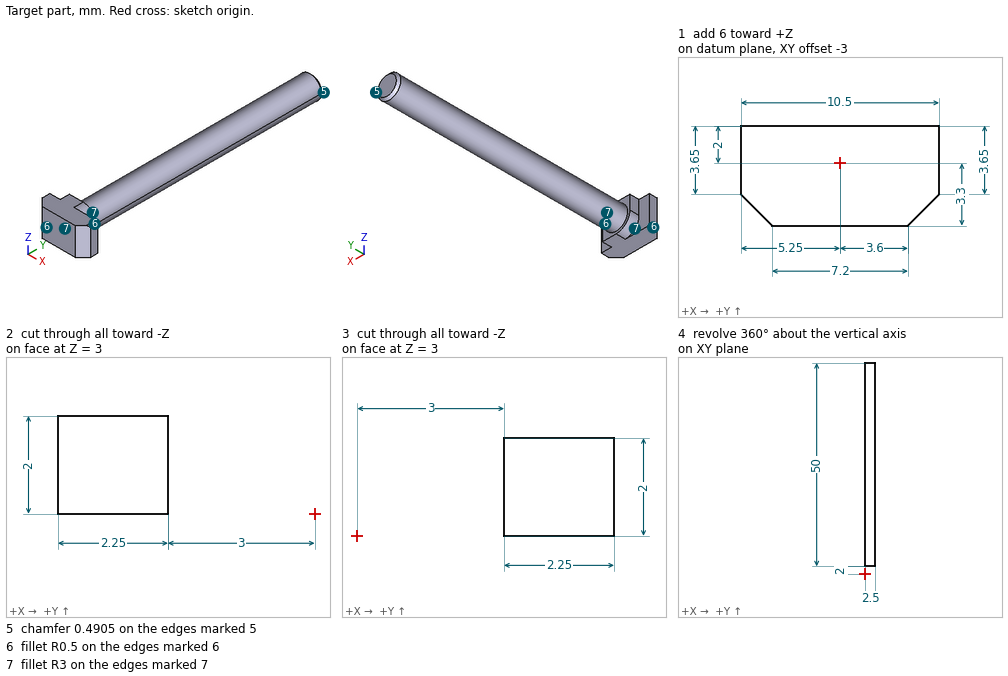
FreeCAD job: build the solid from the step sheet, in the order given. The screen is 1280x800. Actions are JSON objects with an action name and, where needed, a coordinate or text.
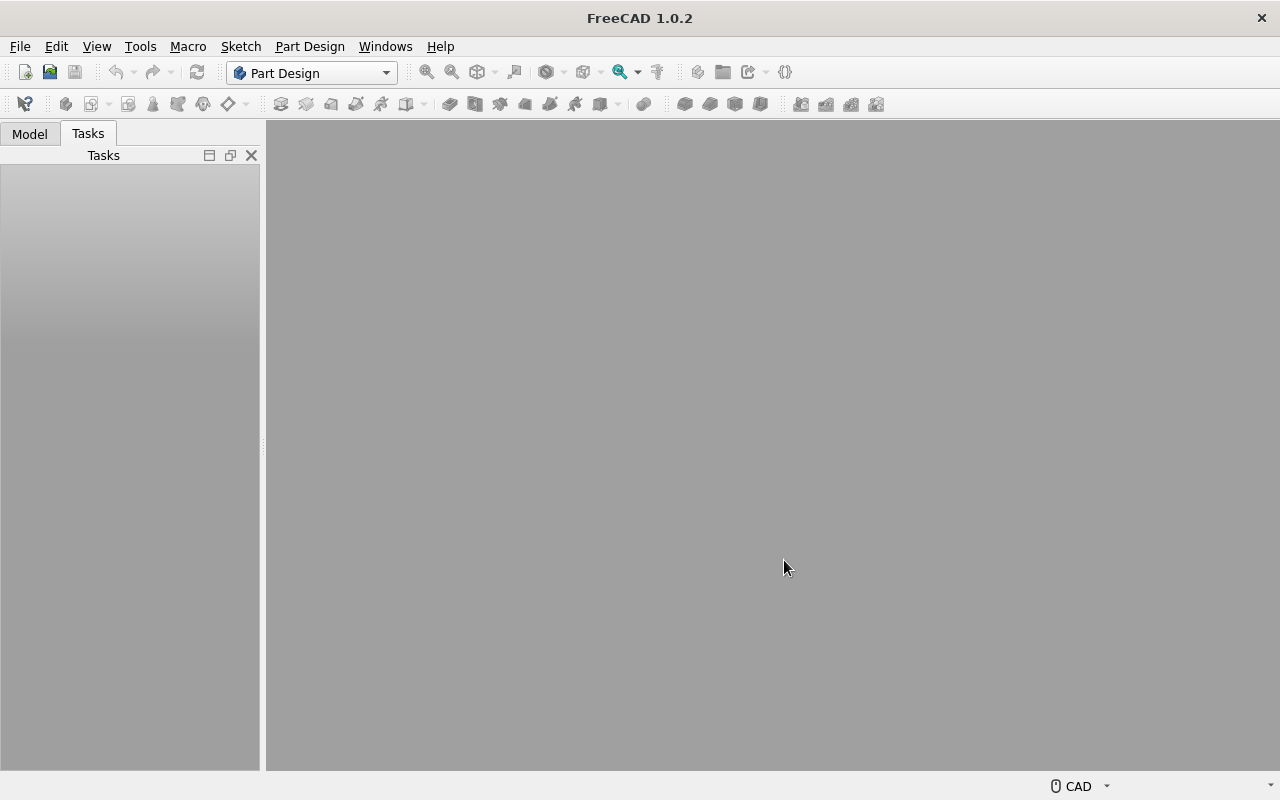
{"action": "key", "text": "ctrl+n"}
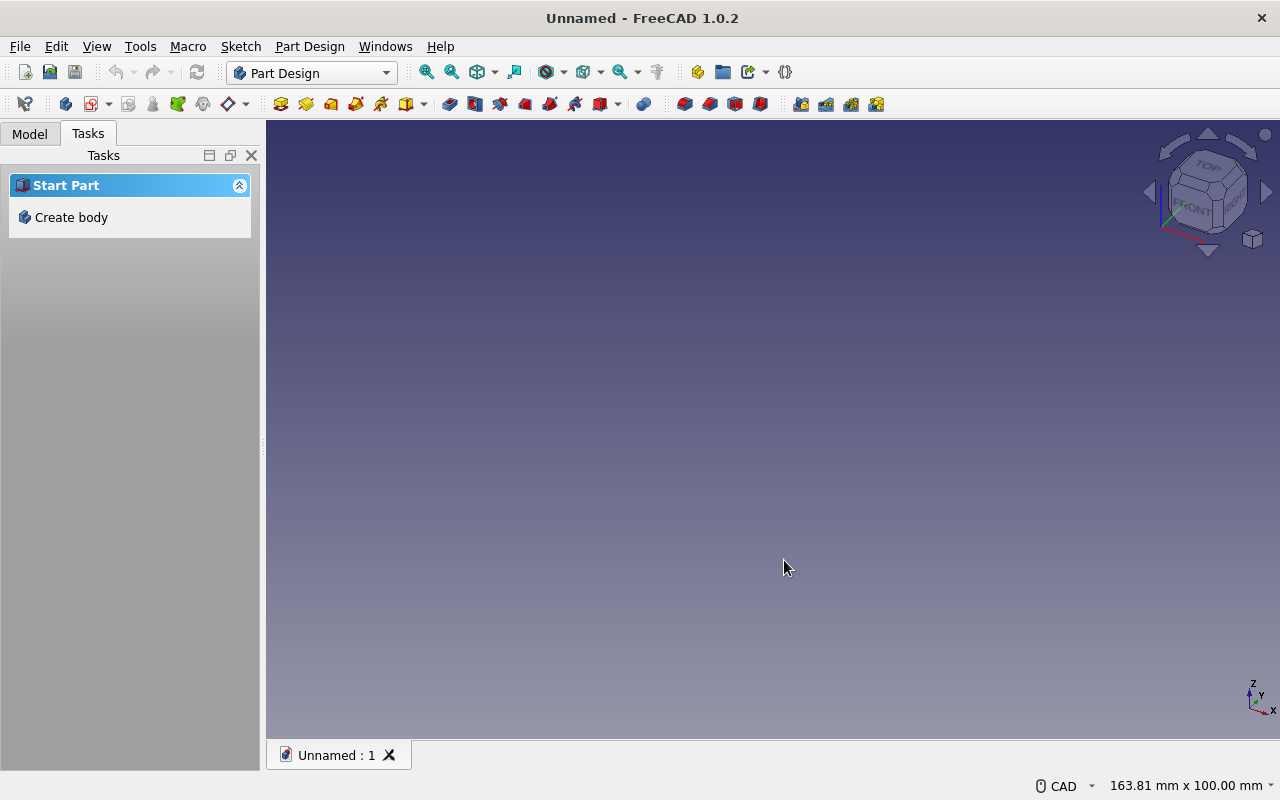
{"action": "left_click", "coordinate": [66, 104]}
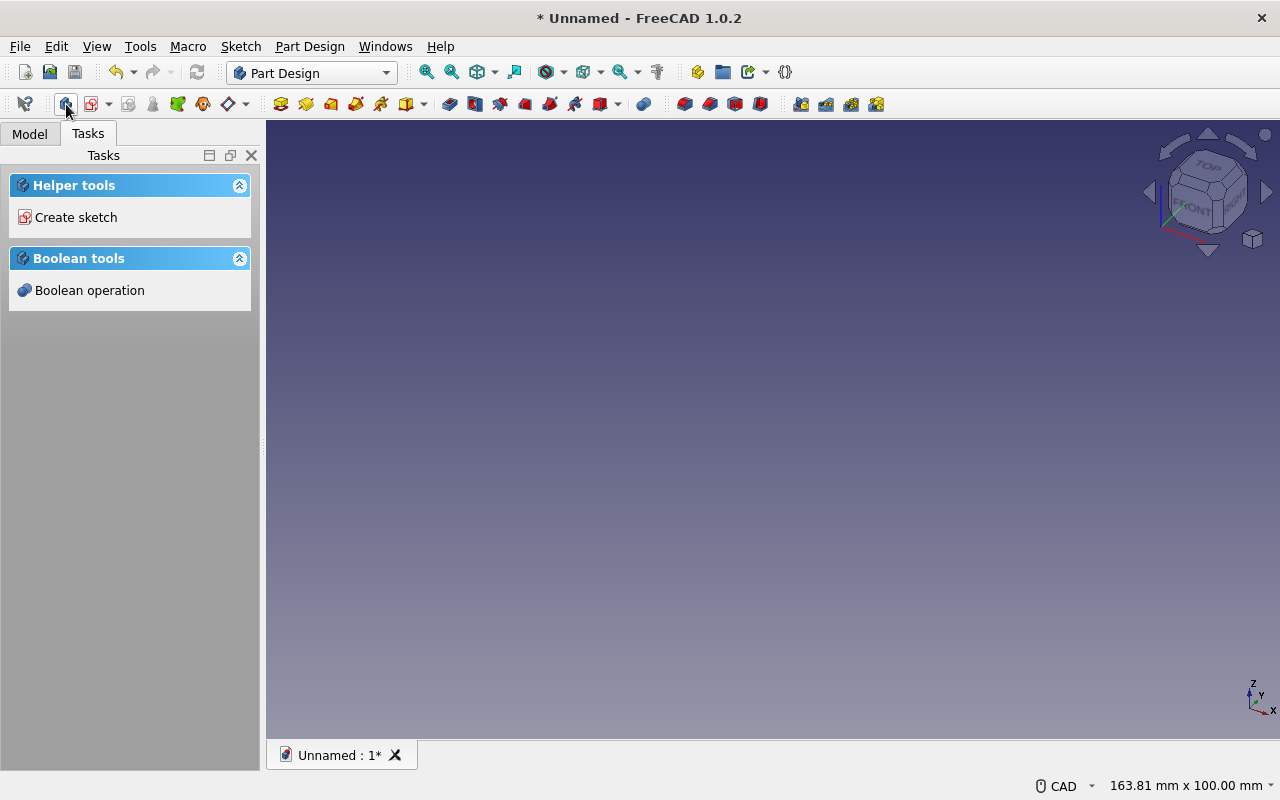
{"action": "left_click", "coordinate": [30, 134]}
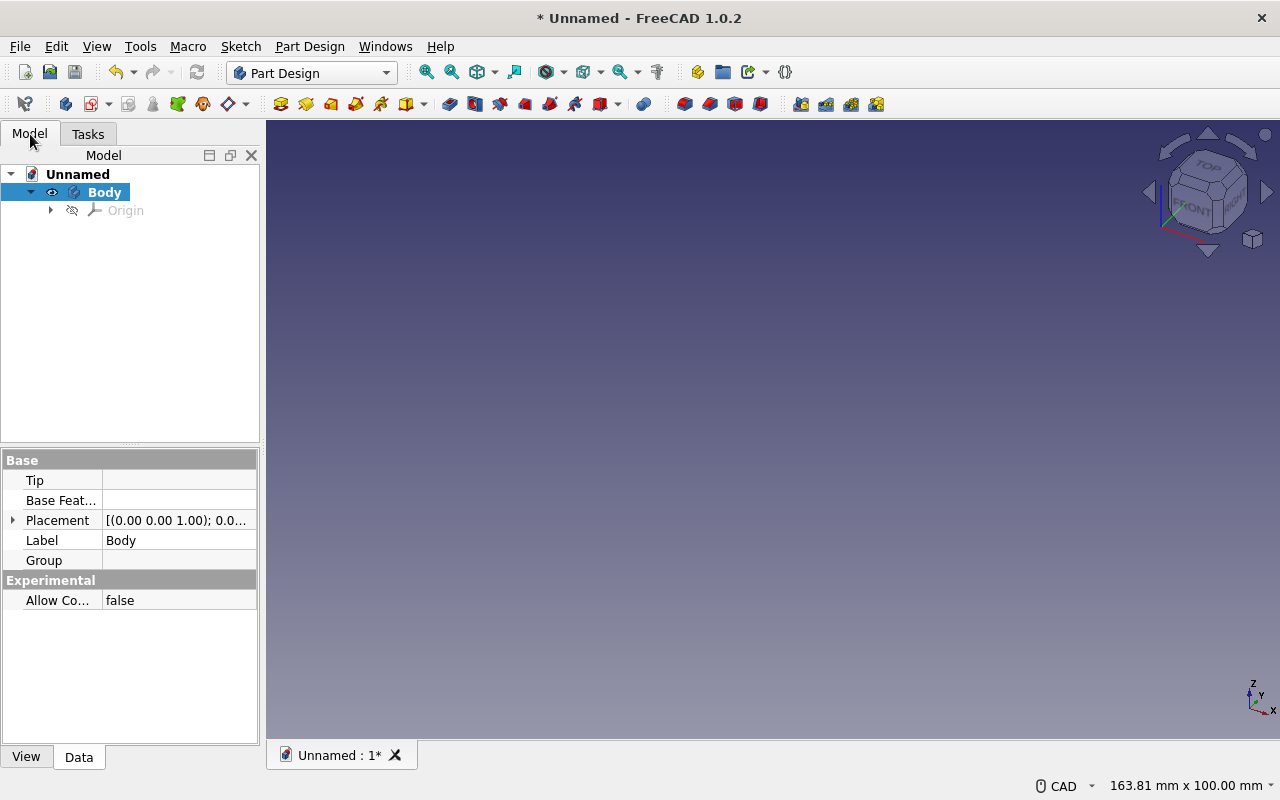
{"action": "left_click", "coordinate": [51, 210]}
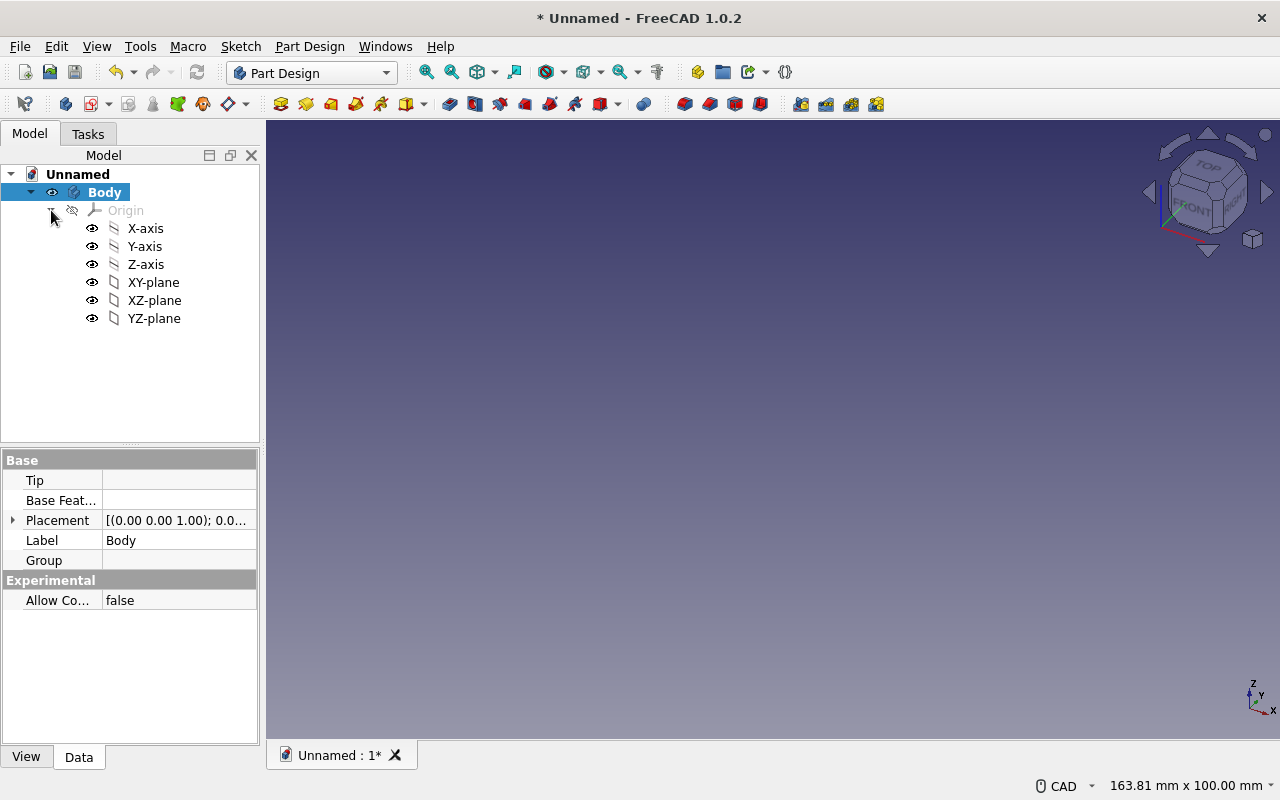
{"action": "left_click", "coordinate": [137, 282]}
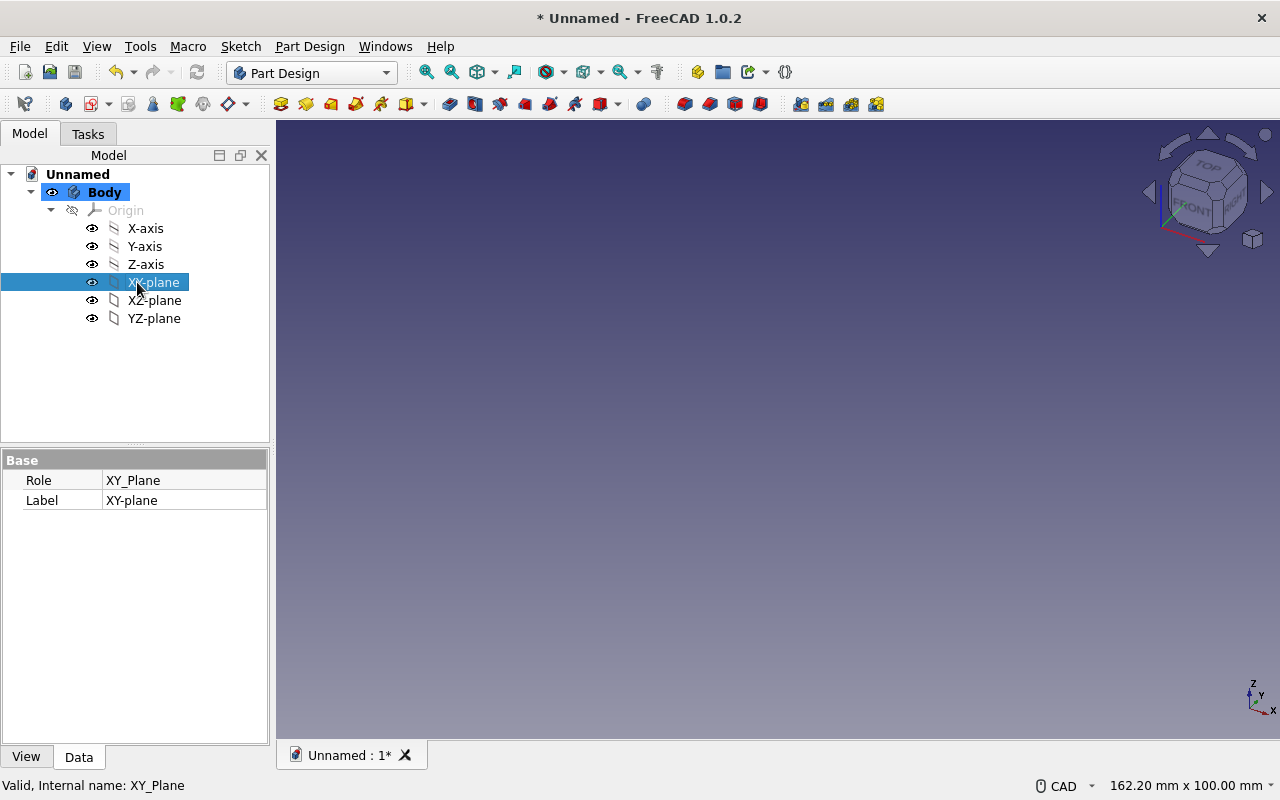
{"action": "left_click", "coordinate": [228, 104]}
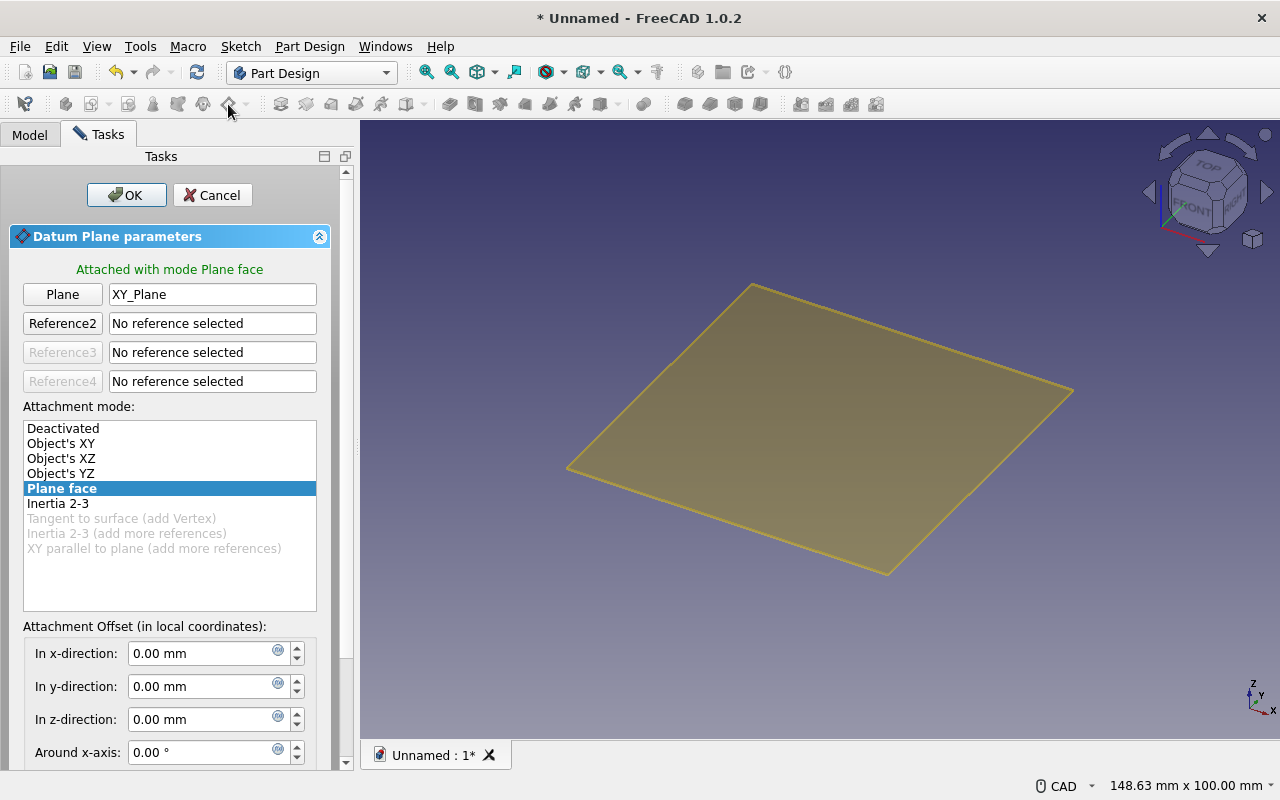
{"action": "triple_click", "coordinate": [210, 720]}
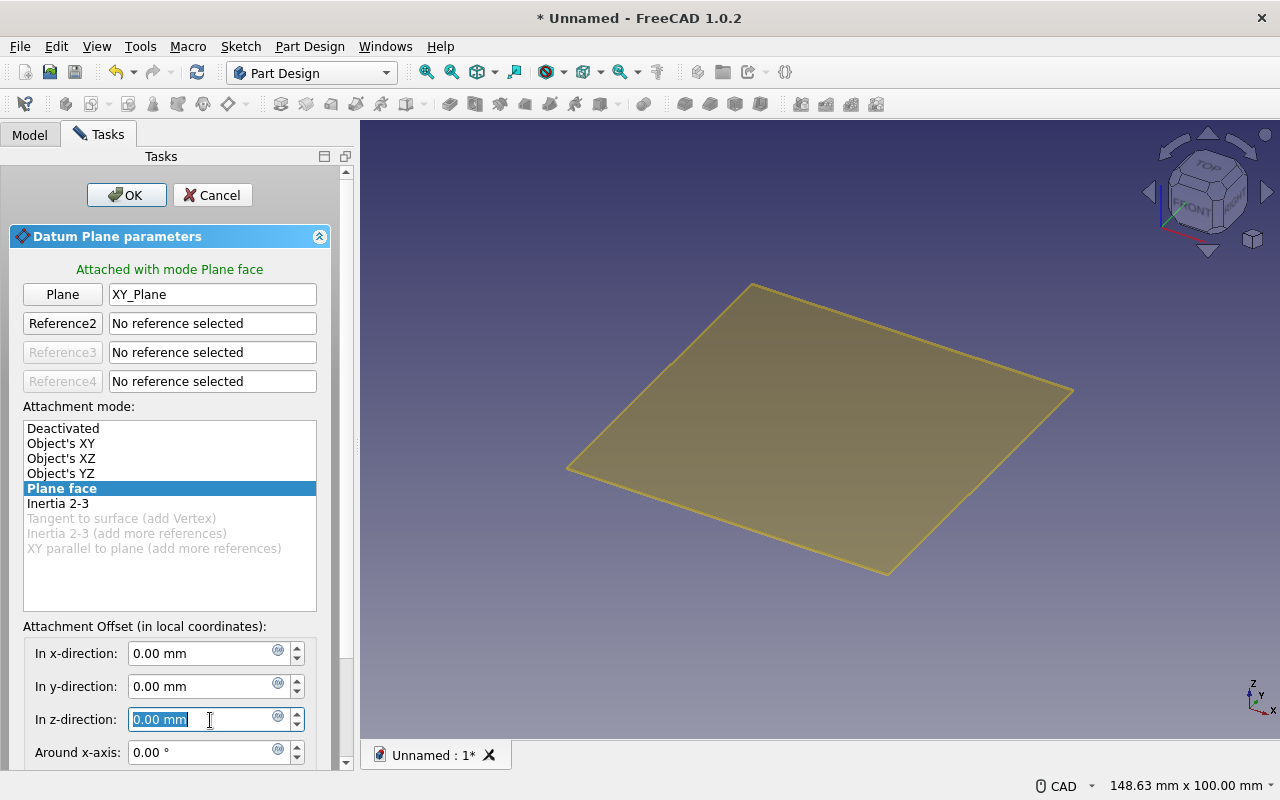
{"action": "type", "text": "-3"}
{"action": "key", "text": "Tab"}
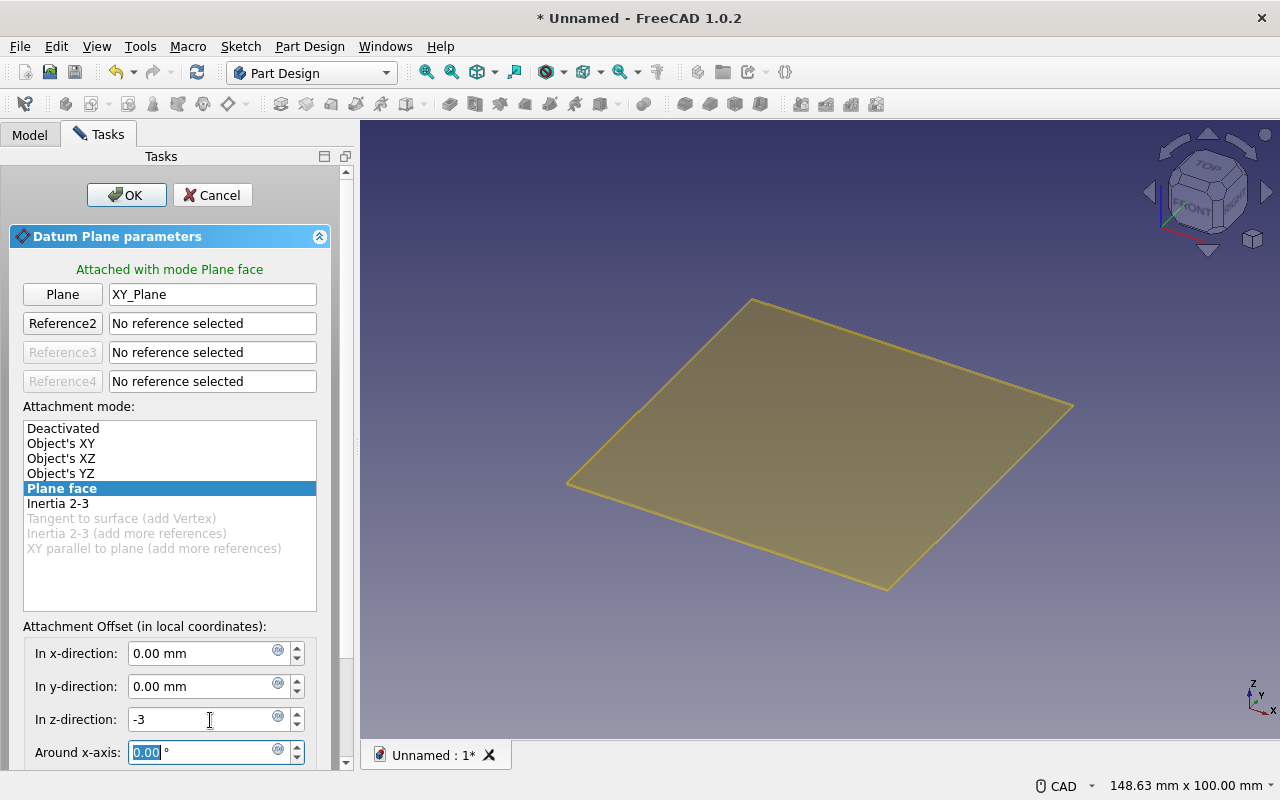
{"action": "left_click", "coordinate": [127, 195]}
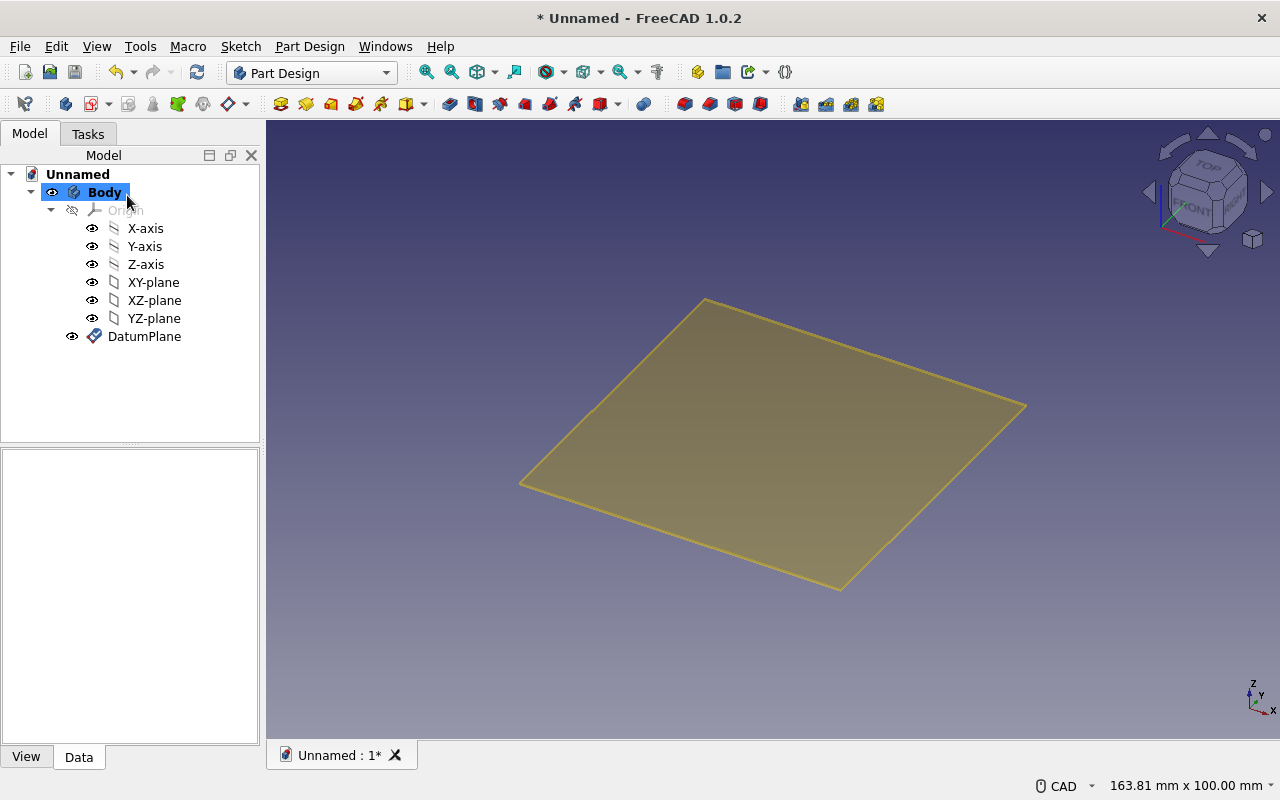
{"action": "left_click", "coordinate": [117, 336]}